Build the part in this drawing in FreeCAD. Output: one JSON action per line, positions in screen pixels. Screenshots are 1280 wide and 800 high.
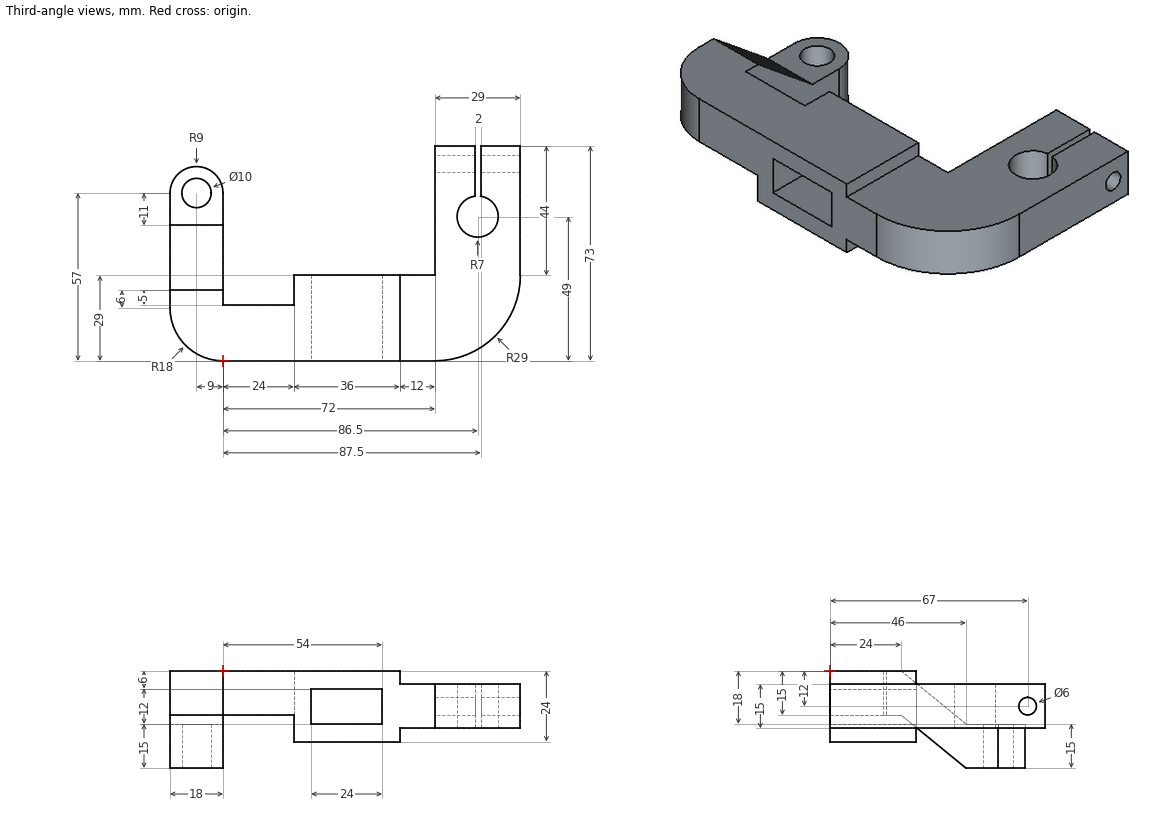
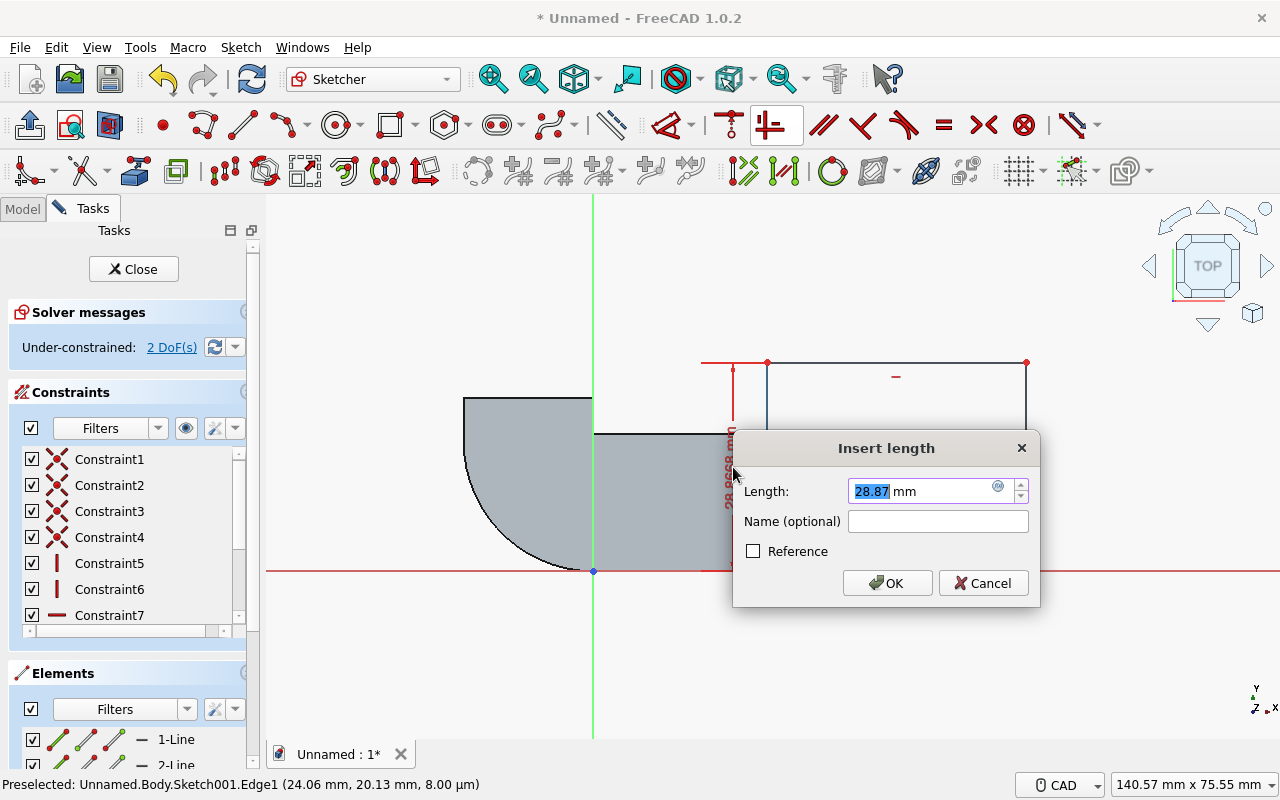
{"action": "type", "text": "29"}
{"action": "key", "text": "Return"}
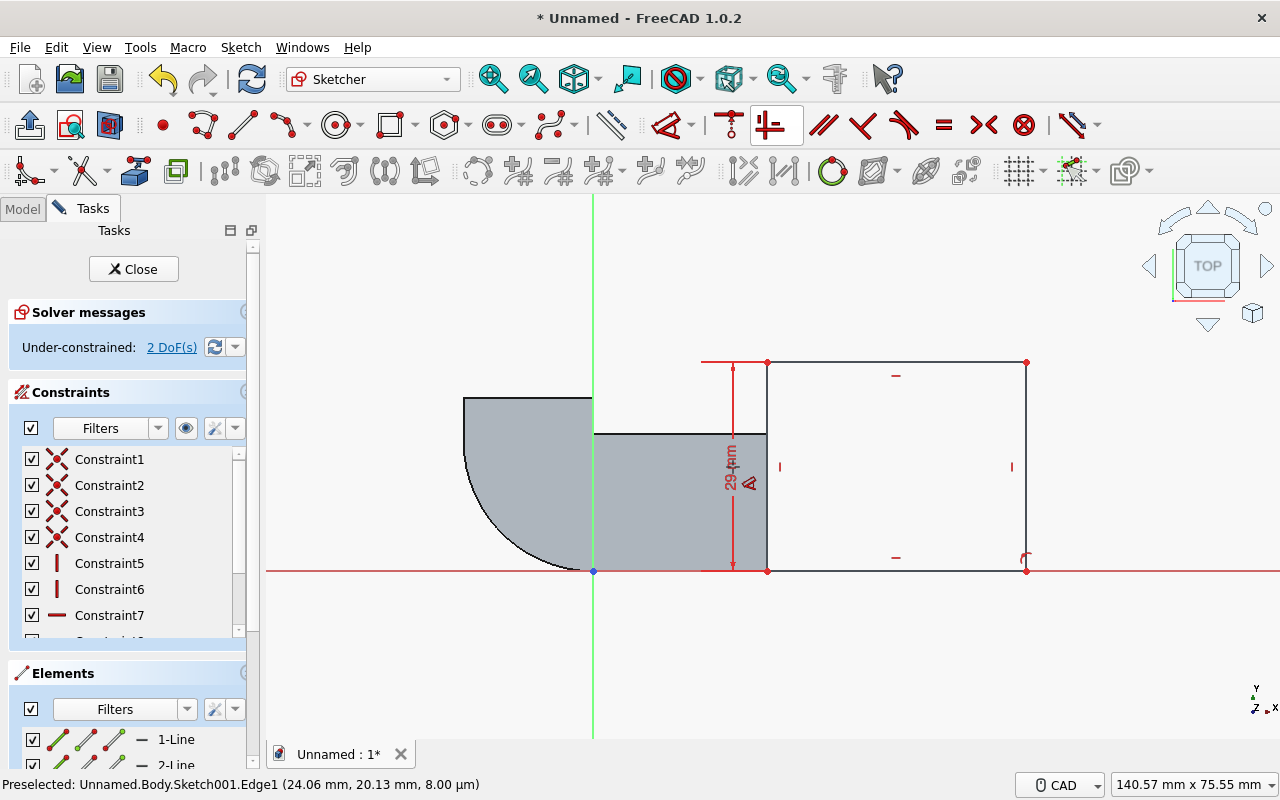
{"action": "left_click", "coordinate": [845, 571]}
{"action": "left_click", "coordinate": [896, 605]}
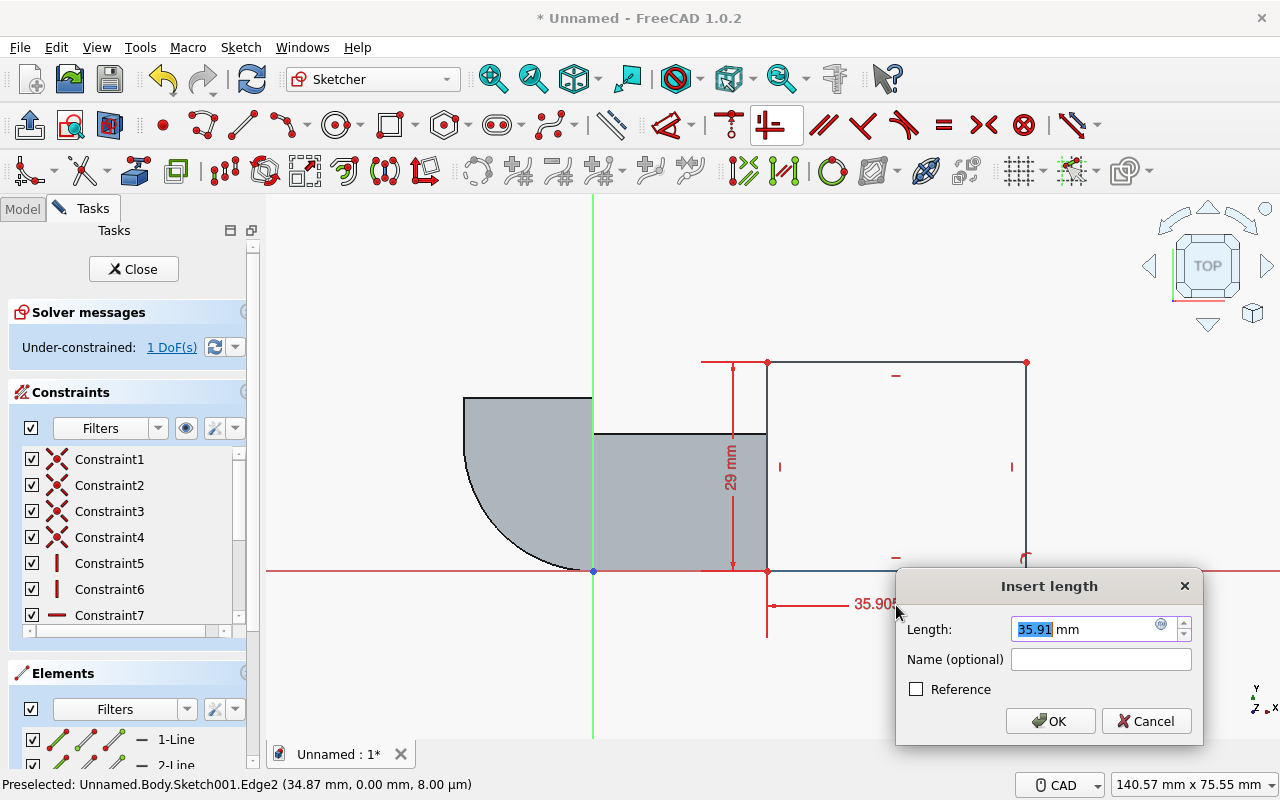
{"action": "type", "text": "36"}
{"action": "key", "text": "Return"}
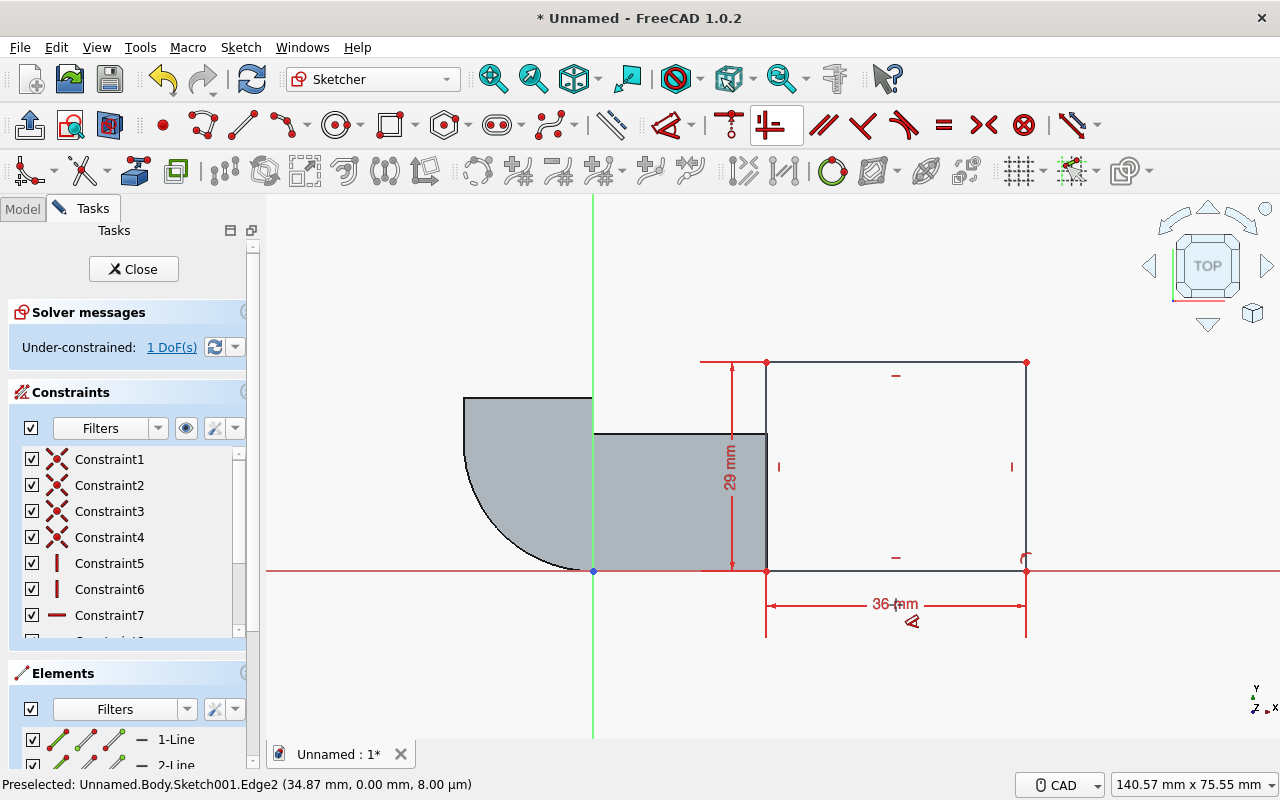
{"action": "left_click", "coordinate": [766, 362]}
{"action": "left_click", "coordinate": [680, 605]}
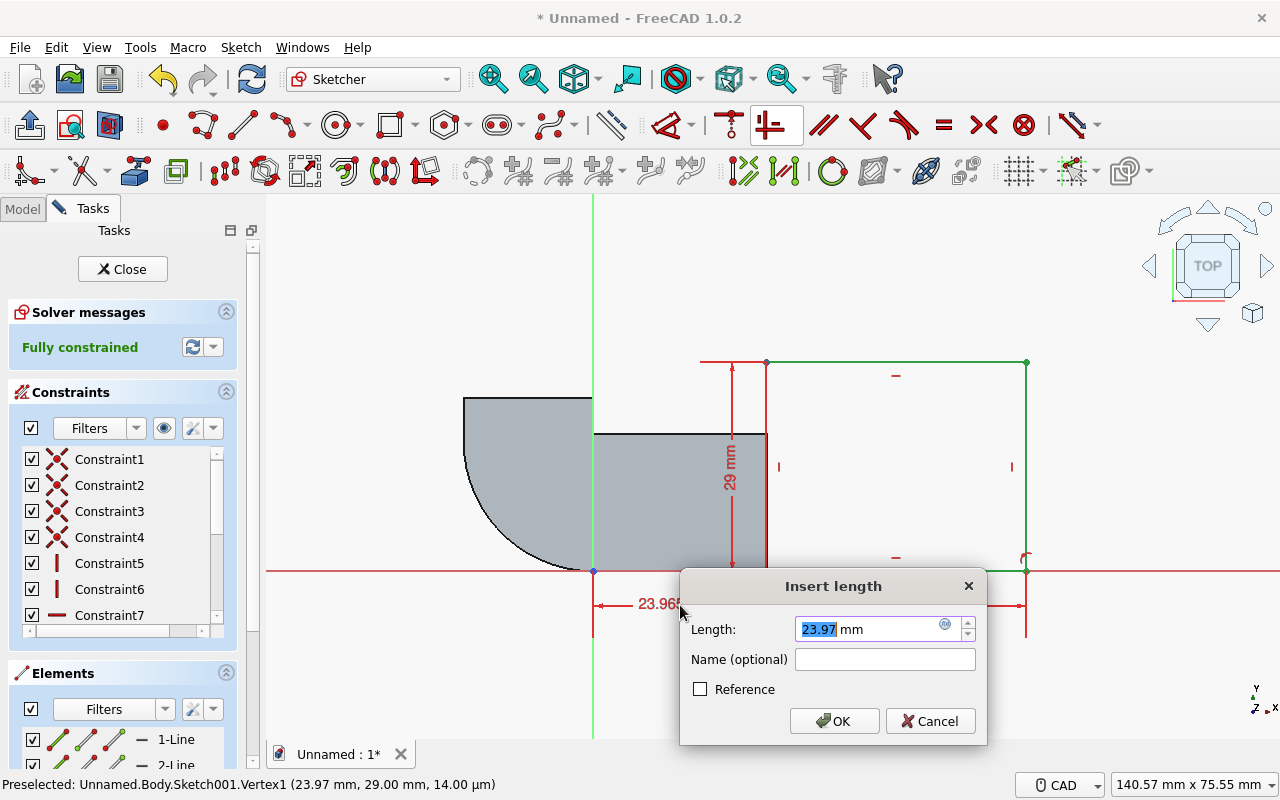
{"action": "type", "text": "24"}
{"action": "key", "text": "Return"}
{"action": "key", "text": "Escape"}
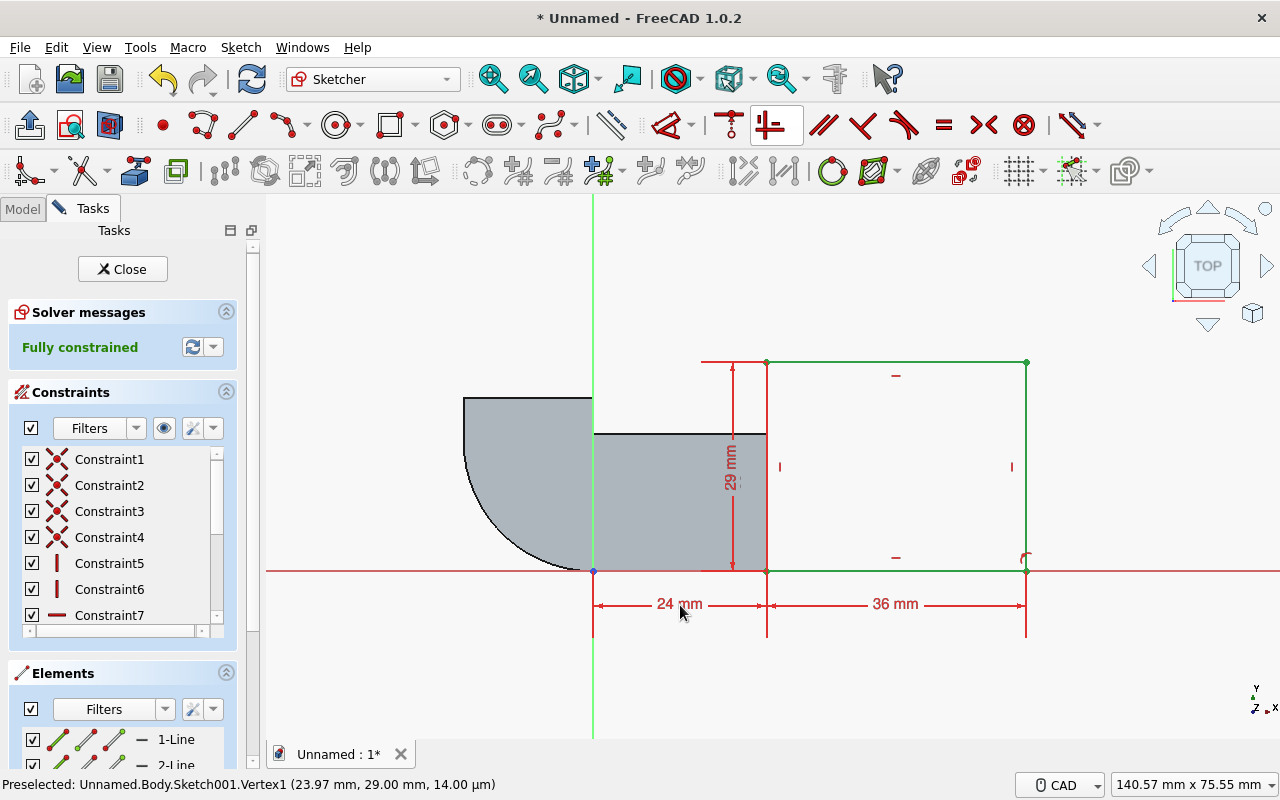
{"action": "left_click", "coordinate": [123, 269]}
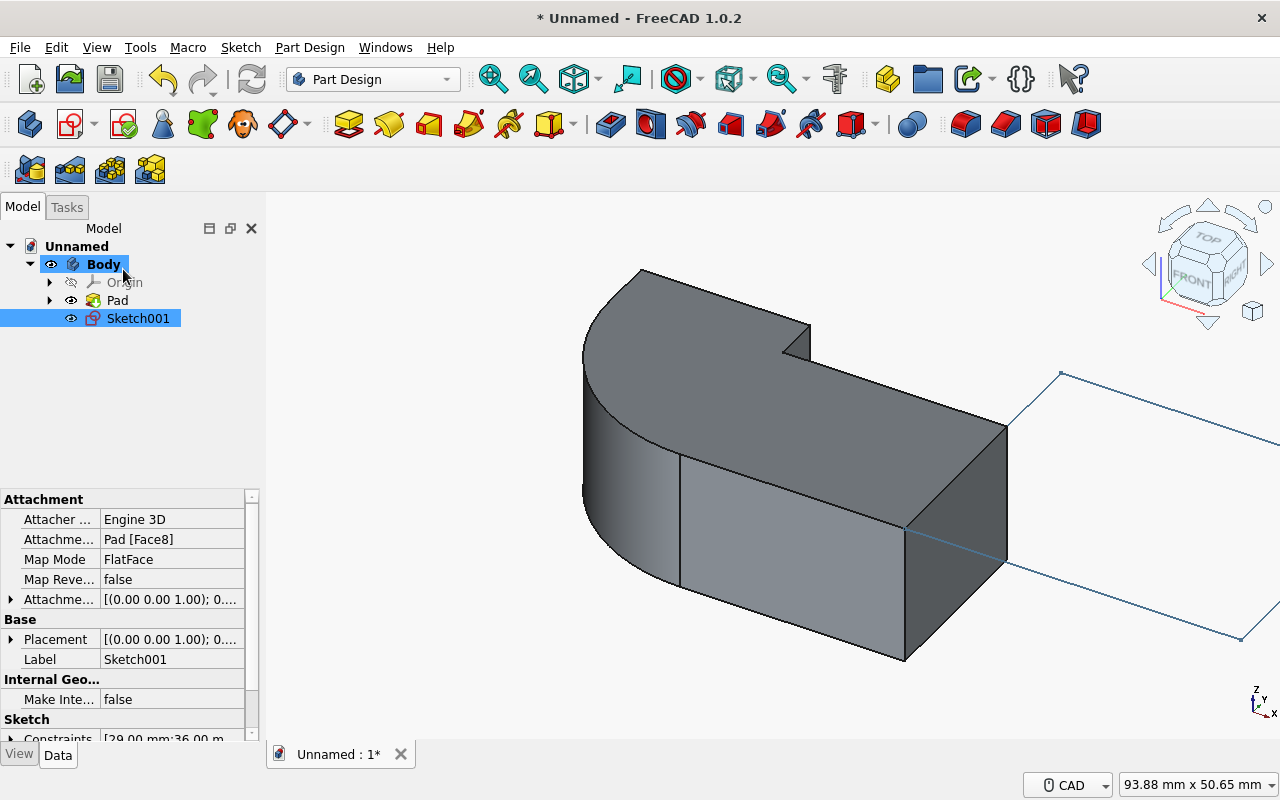
{"action": "left_click", "coordinate": [350, 124]}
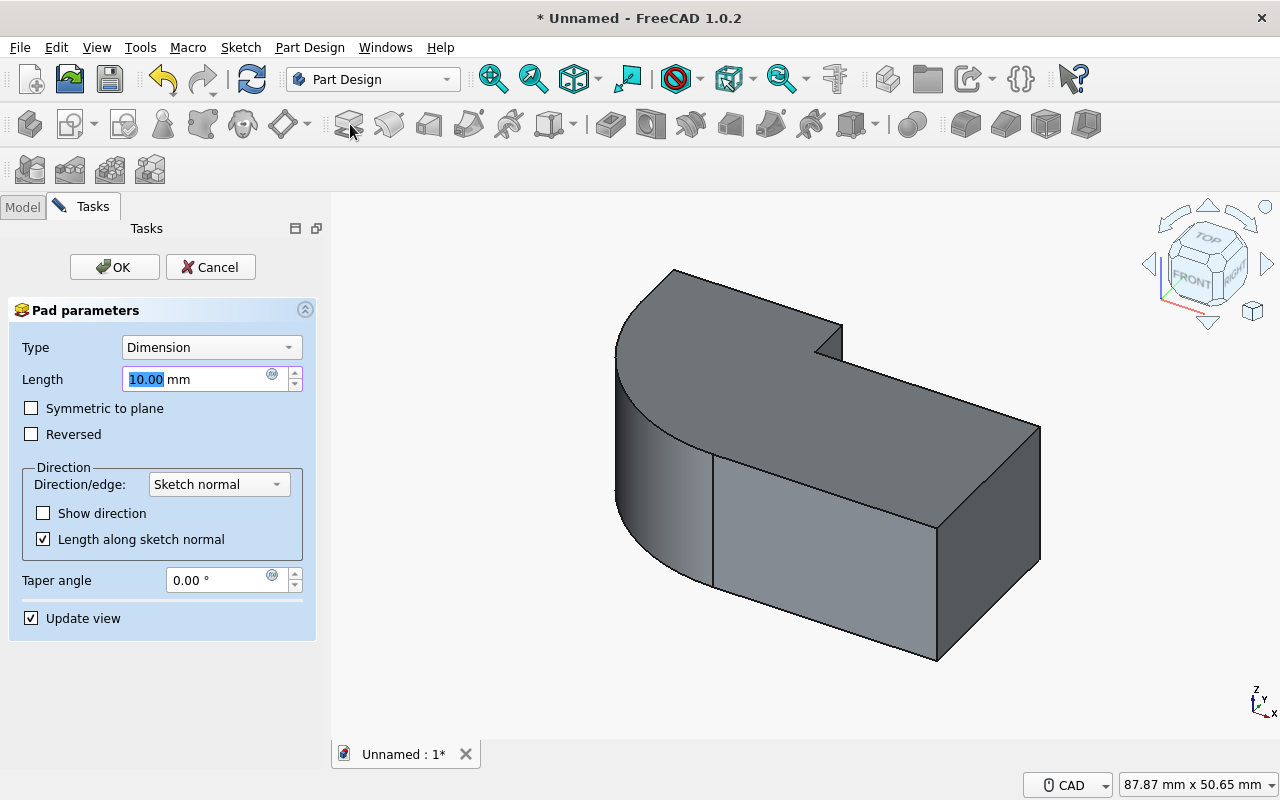
{"action": "type", "text": "24"}
{"action": "key", "text": "Tab"}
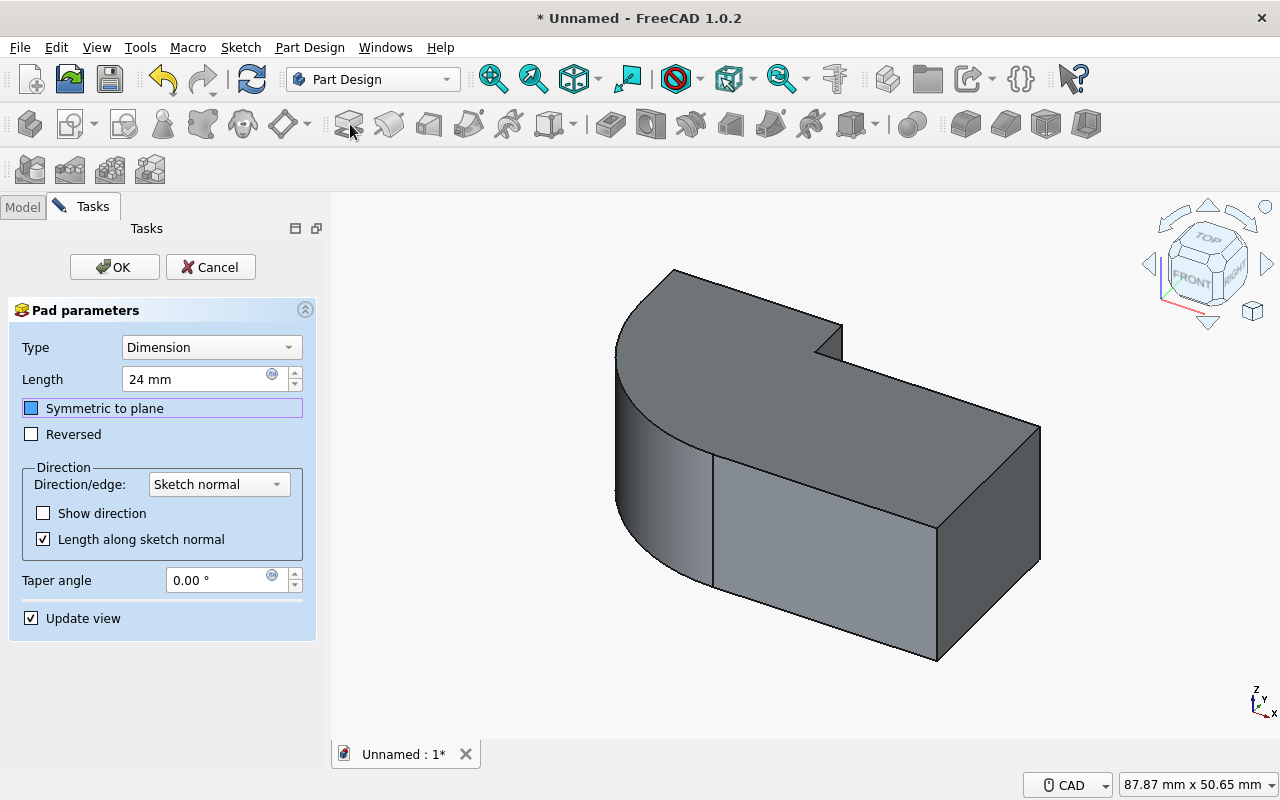
{"action": "left_click", "coordinate": [30, 434]}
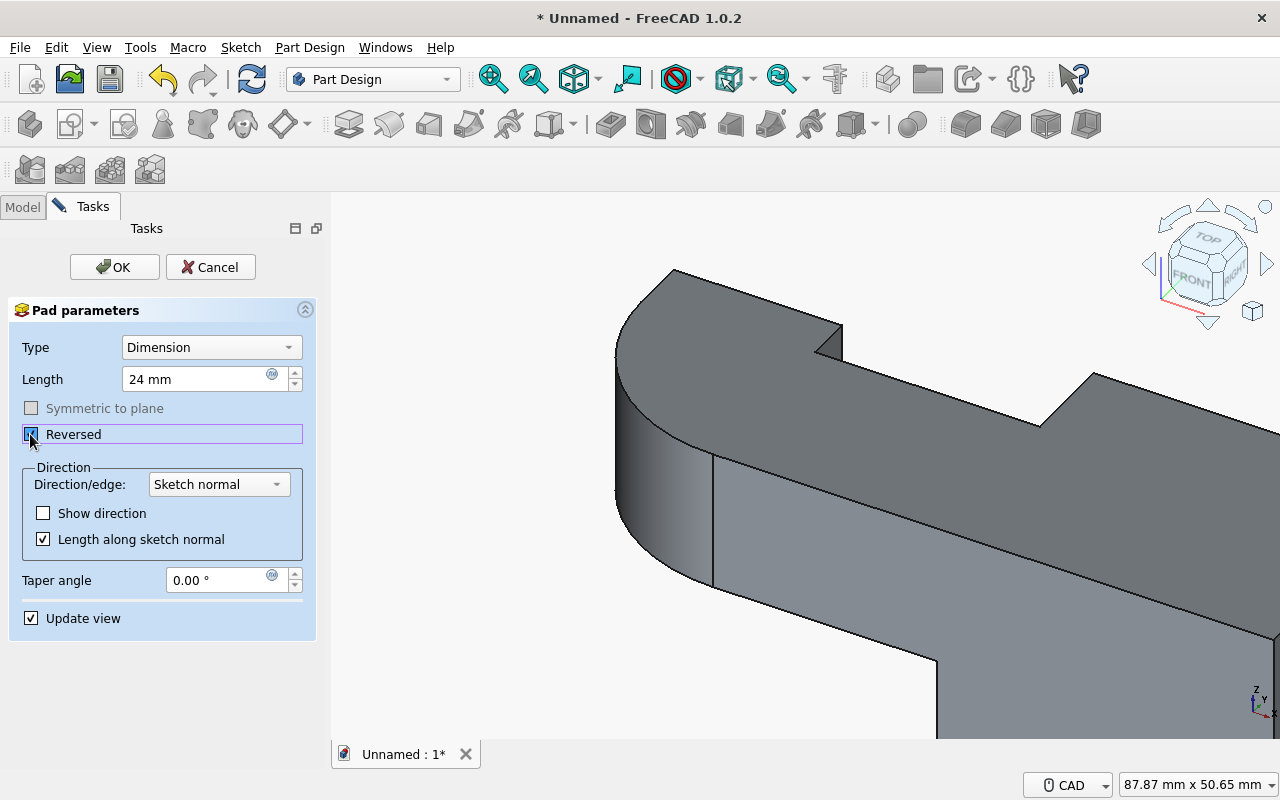
{"action": "left_click", "coordinate": [115, 267]}